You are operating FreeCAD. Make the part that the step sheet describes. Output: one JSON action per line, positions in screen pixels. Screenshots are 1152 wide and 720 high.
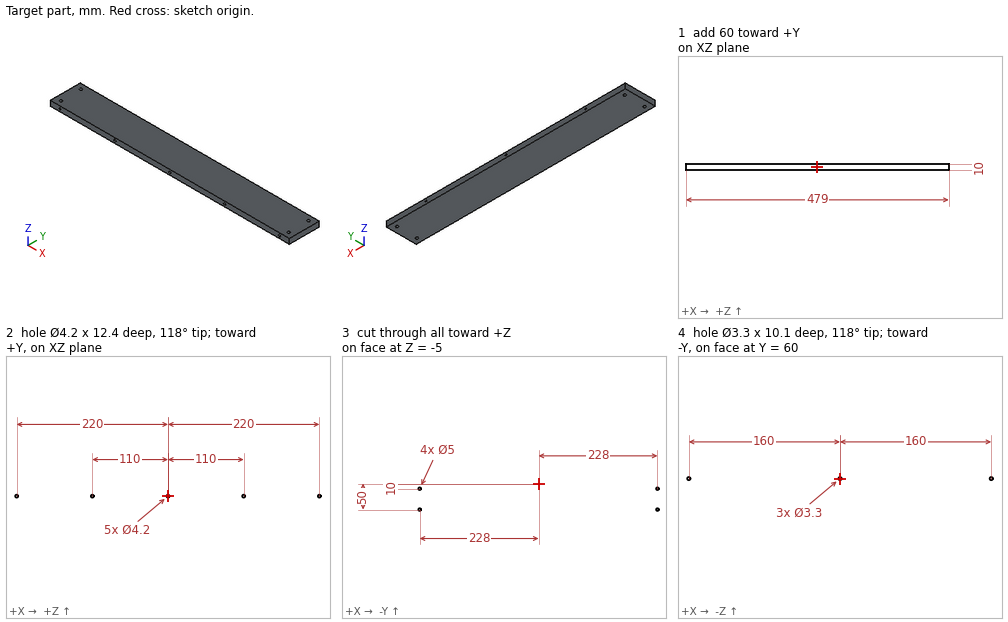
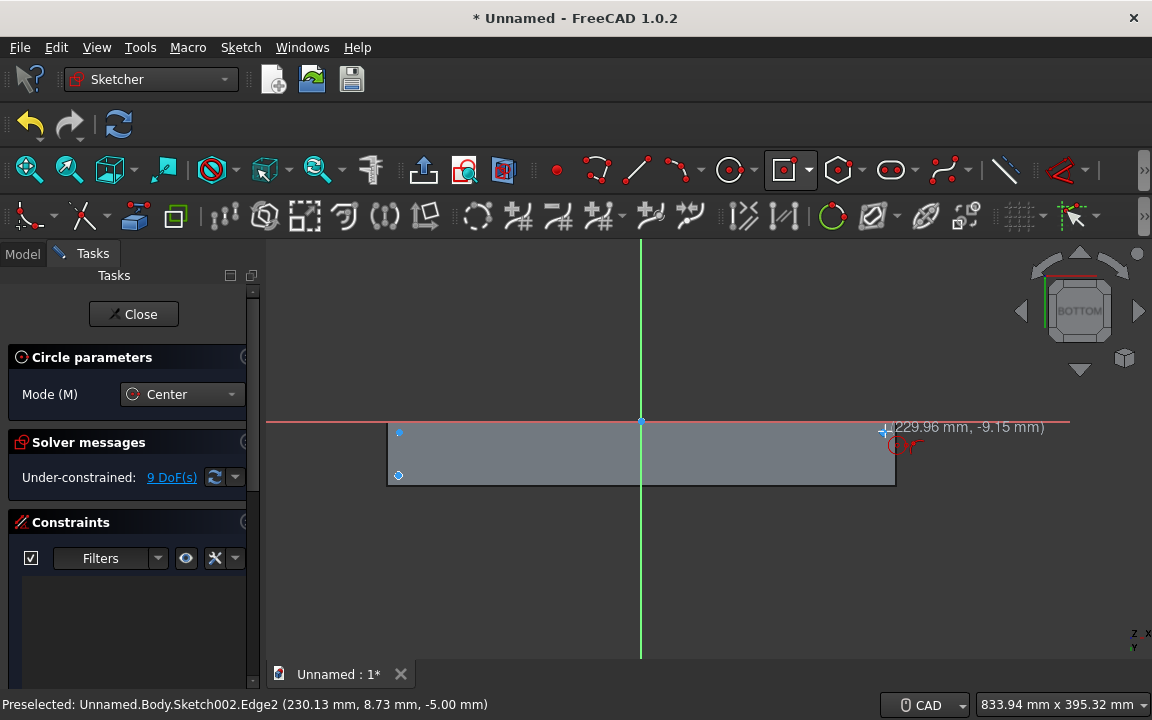
{"action": "scroll", "coordinate": [883, 475], "scroll_direction": "up", "scroll_amount": 11}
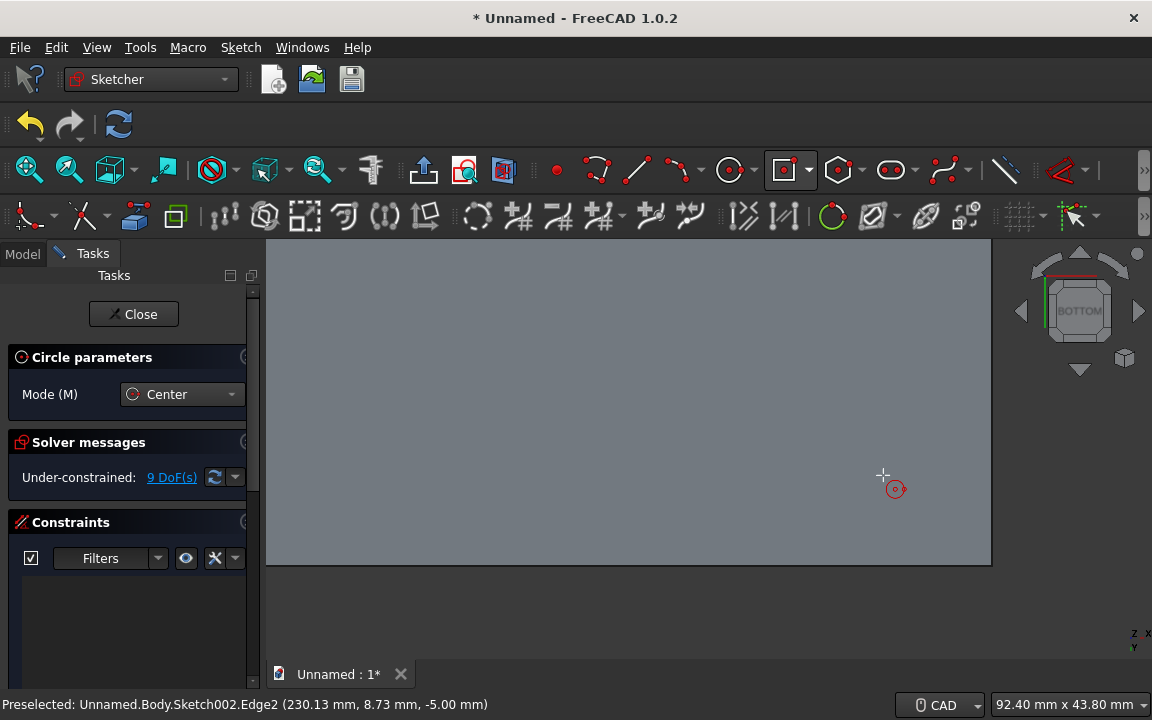
{"action": "scroll", "coordinate": [883, 475], "scroll_direction": "down", "scroll_amount": 11}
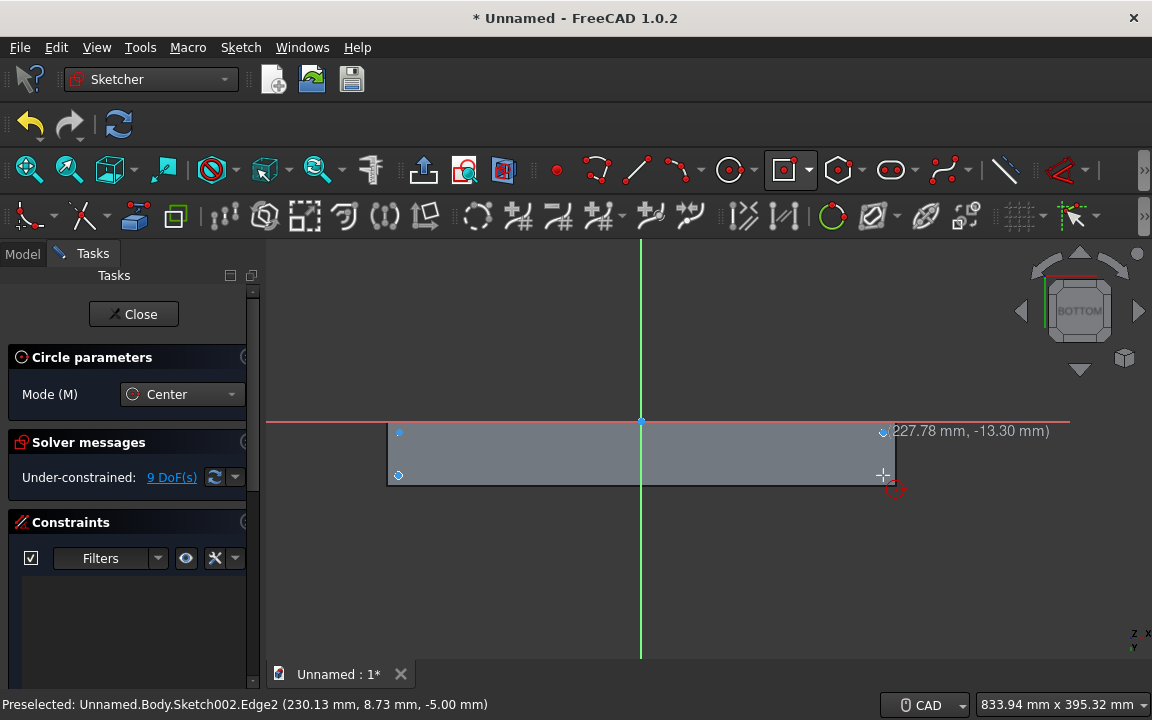
{"action": "left_click", "coordinate": [883, 475]}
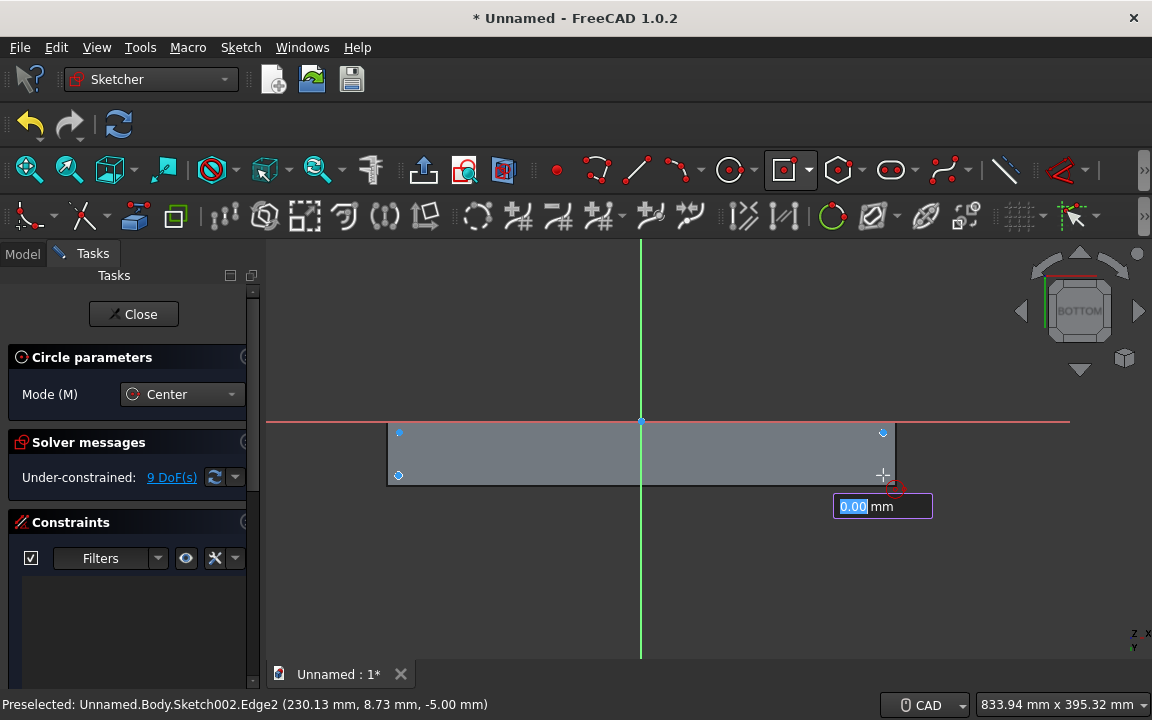
{"action": "scroll", "coordinate": [885, 473], "scroll_direction": "up", "scroll_amount": 9}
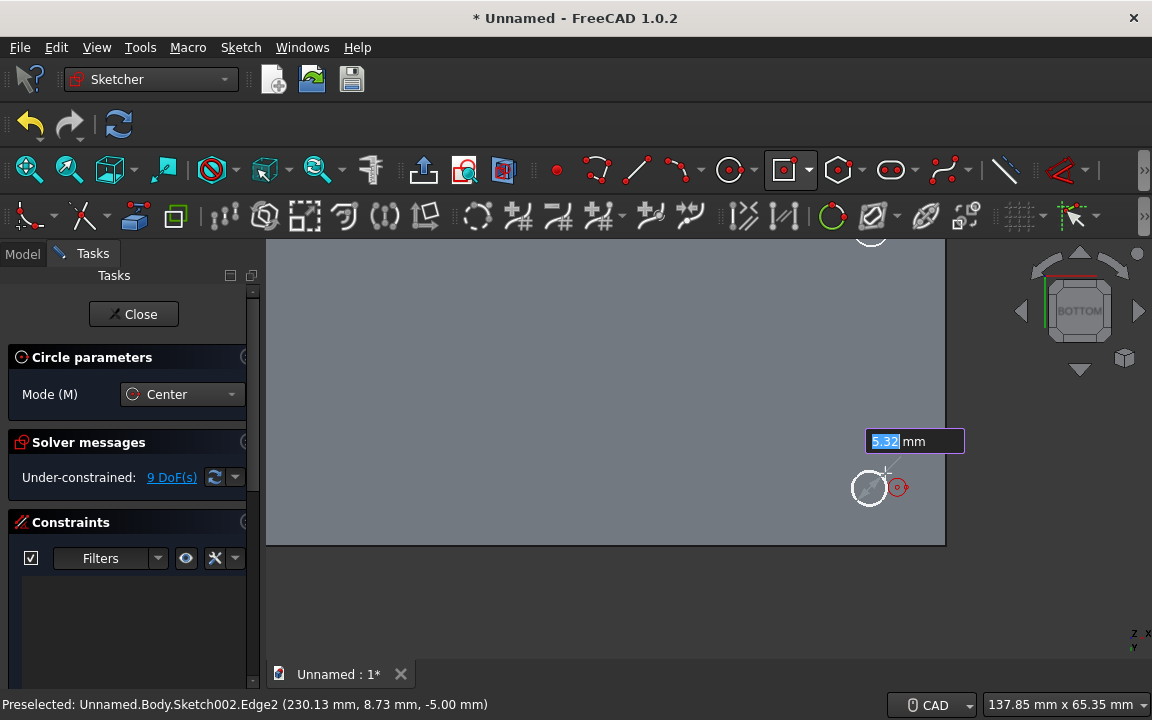
{"action": "left_click", "coordinate": [884, 471]}
{"action": "key", "text": "Escape"}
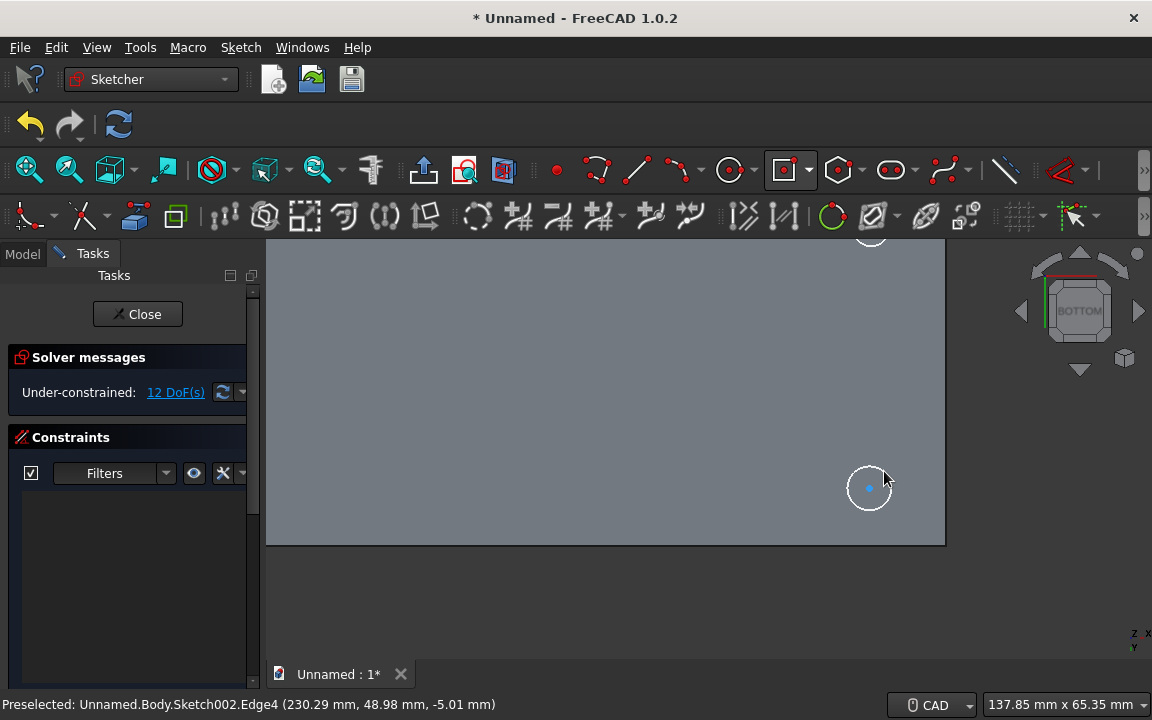
{"action": "scroll", "coordinate": [885, 473], "scroll_direction": "down", "scroll_amount": 9}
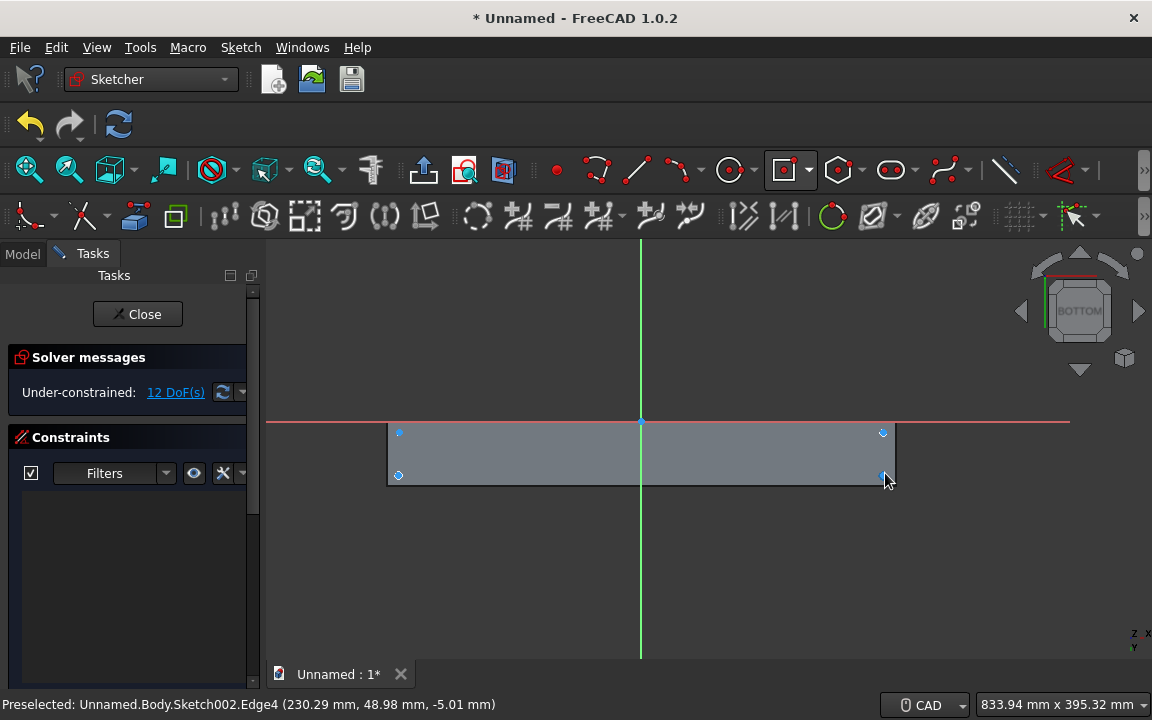
{"action": "scroll", "coordinate": [401, 473], "scroll_direction": "up", "scroll_amount": 8}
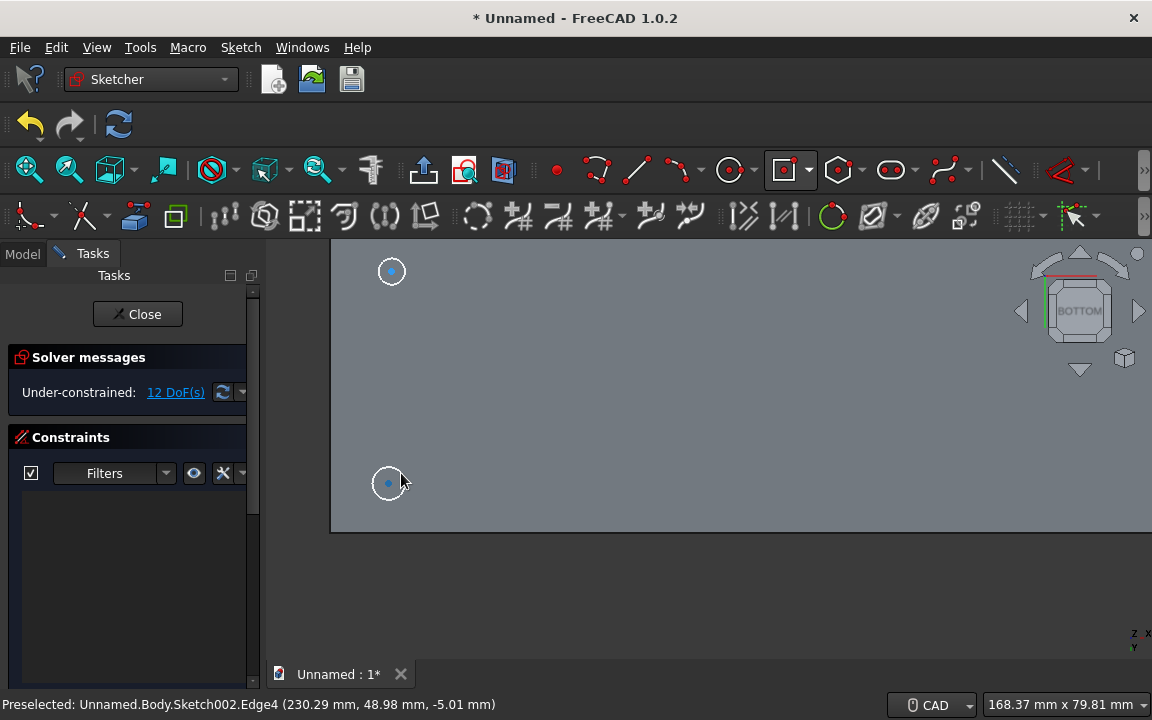
{"action": "left_click", "coordinate": [400, 472]}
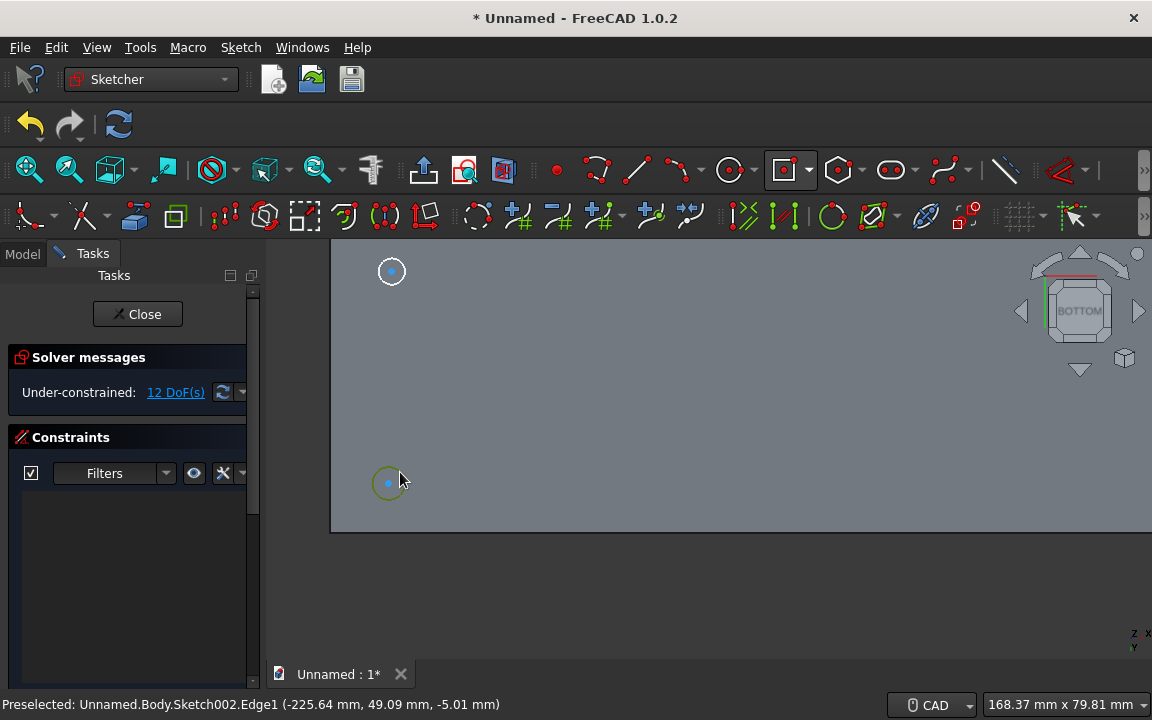
{"action": "left_click", "coordinate": [383, 281]}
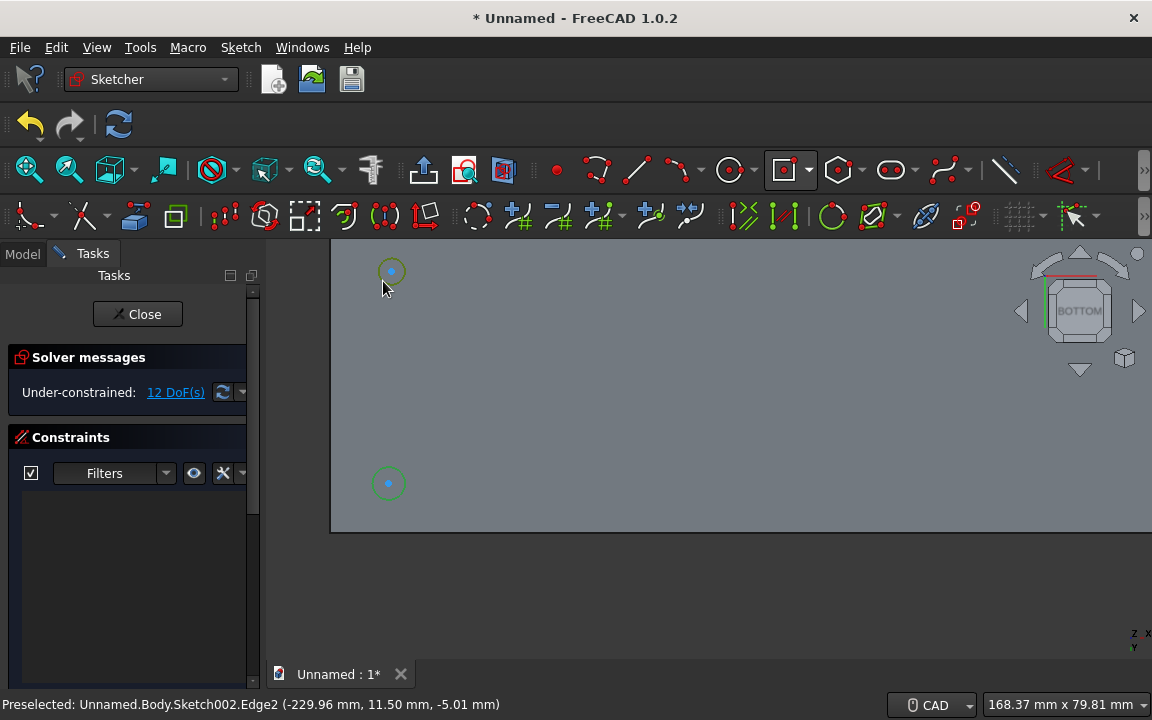
{"action": "scroll", "coordinate": [400, 473], "scroll_direction": "down", "scroll_amount": 8}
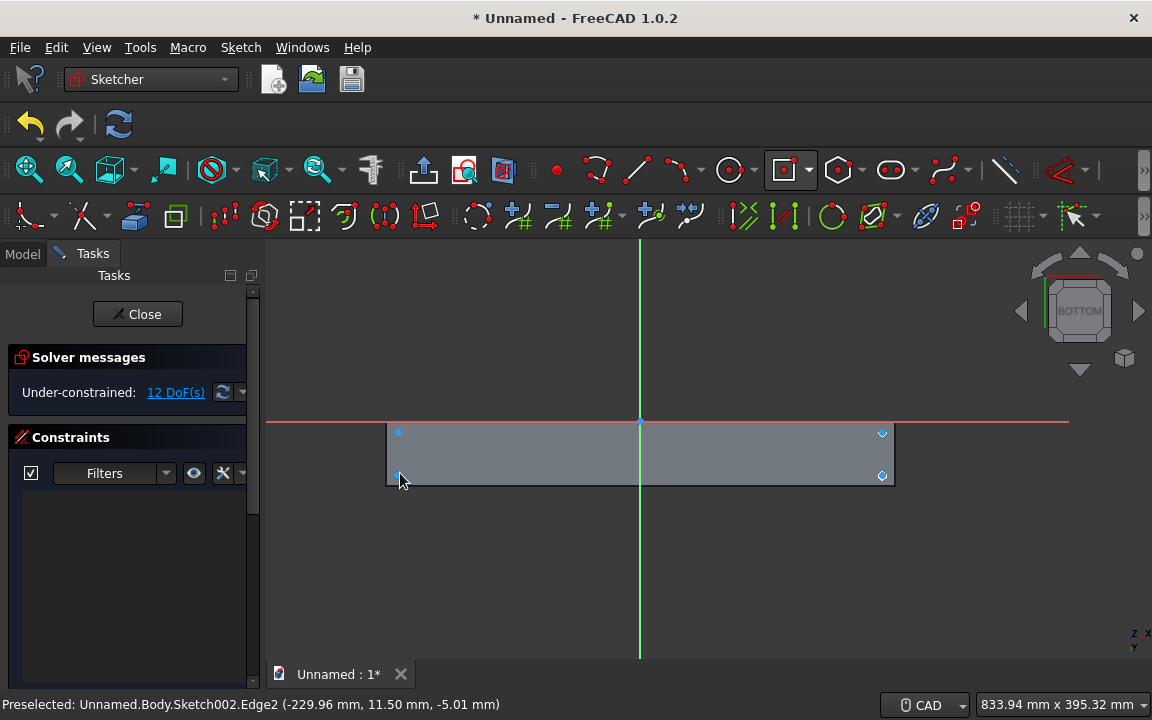
{"action": "scroll", "coordinate": [885, 431], "scroll_direction": "up", "scroll_amount": 8}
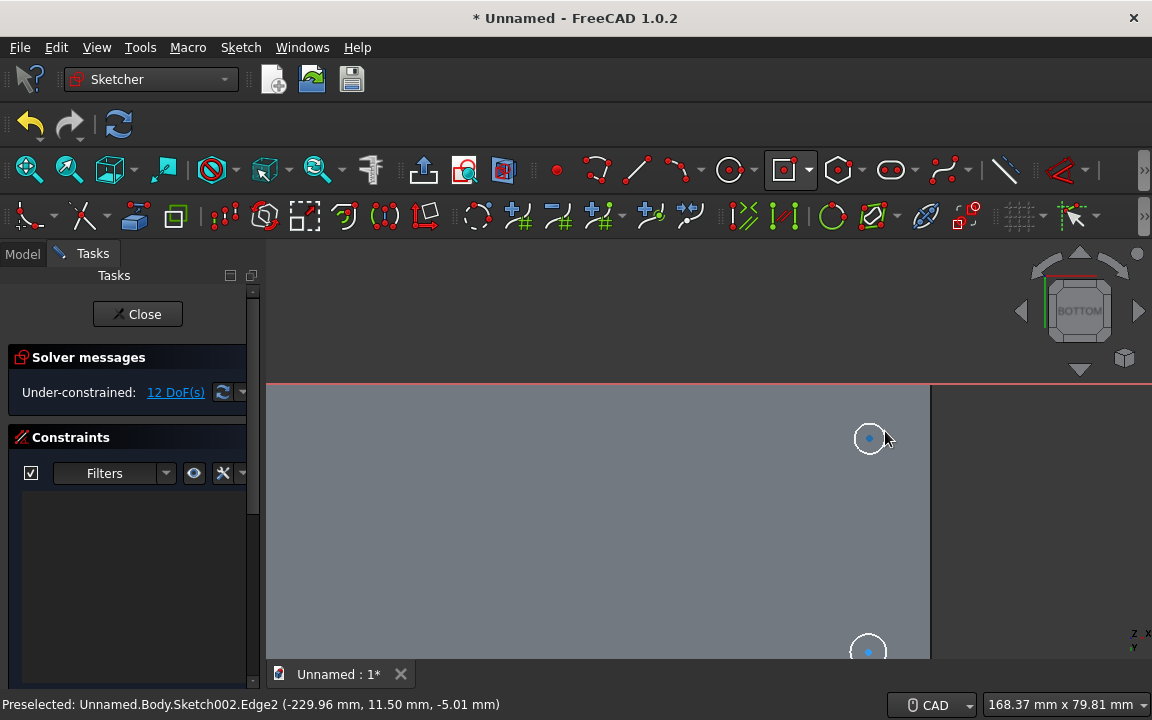
{"action": "left_click", "coordinate": [880, 428]}